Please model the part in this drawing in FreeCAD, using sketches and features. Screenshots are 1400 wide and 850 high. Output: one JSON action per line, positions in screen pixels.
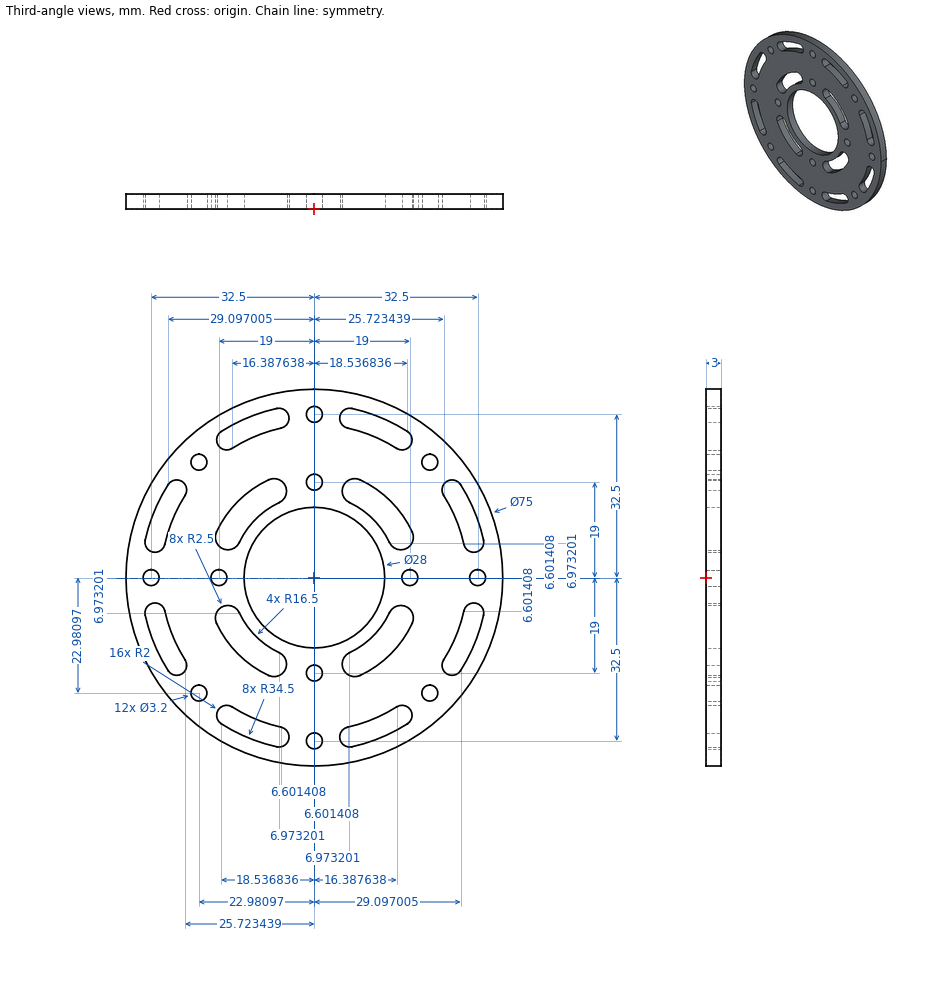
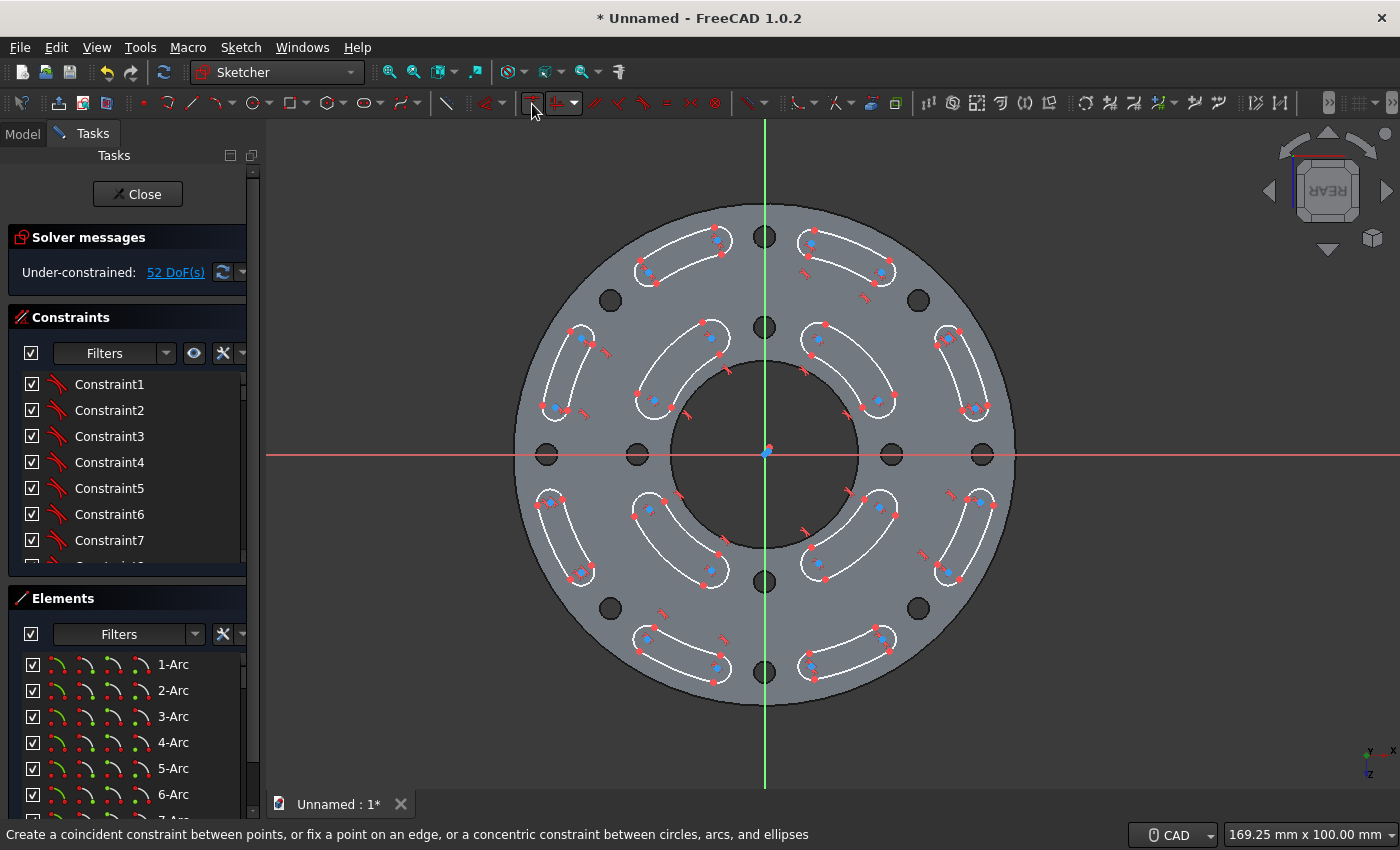
{"action": "left_click", "coordinate": [691, 235]}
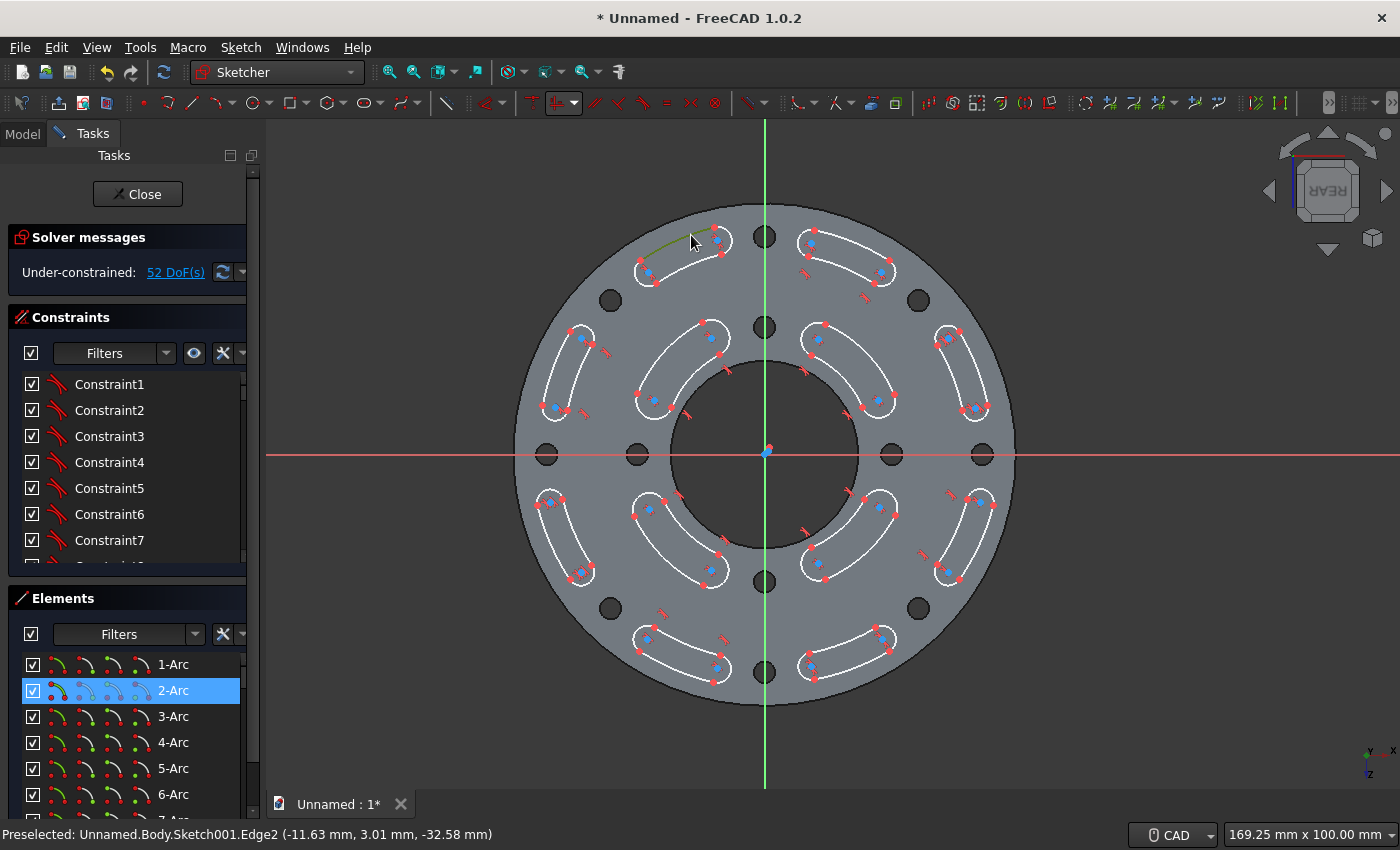
{"action": "left_click", "coordinate": [650, 542]}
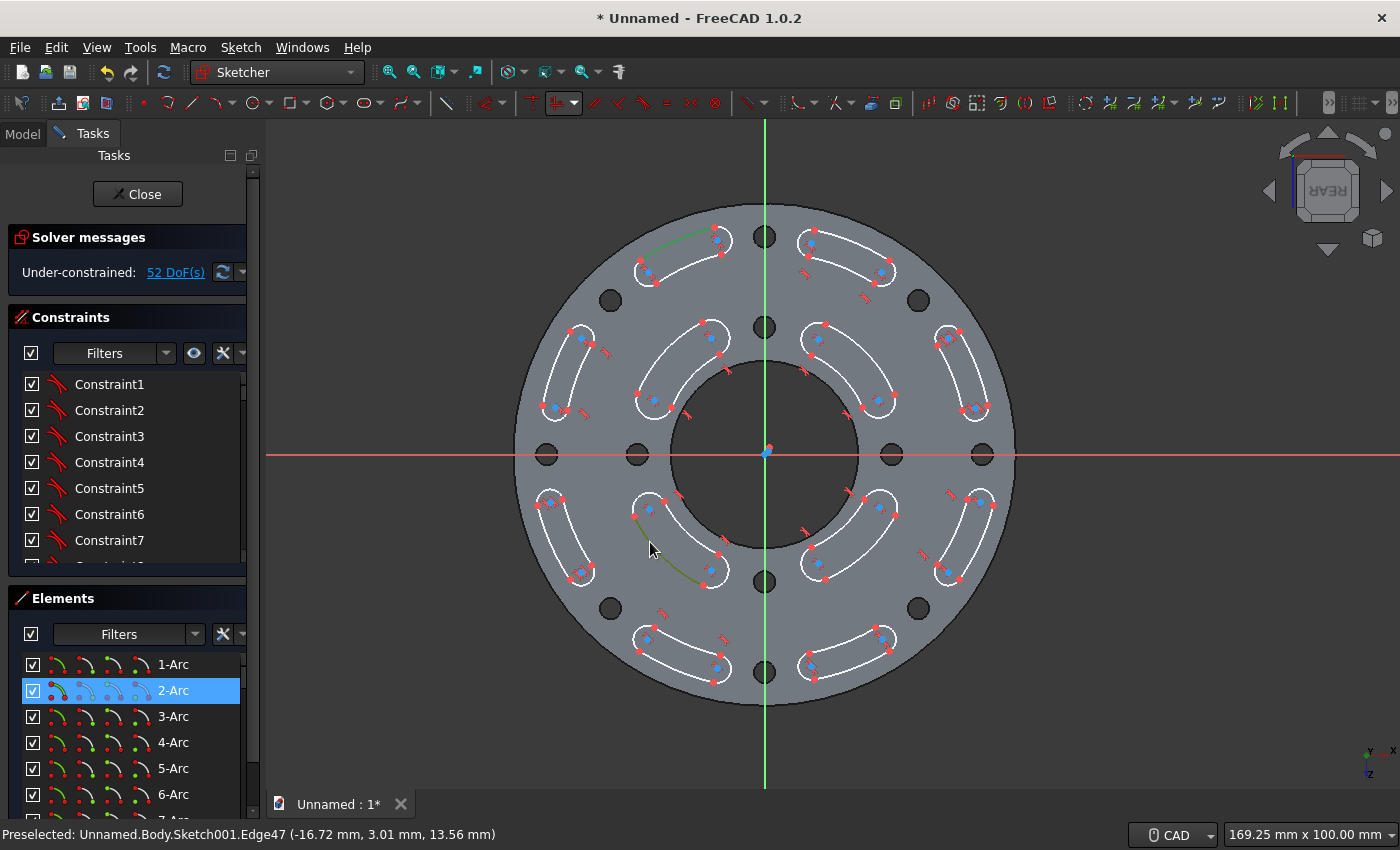
{"action": "left_click", "coordinate": [532, 104]}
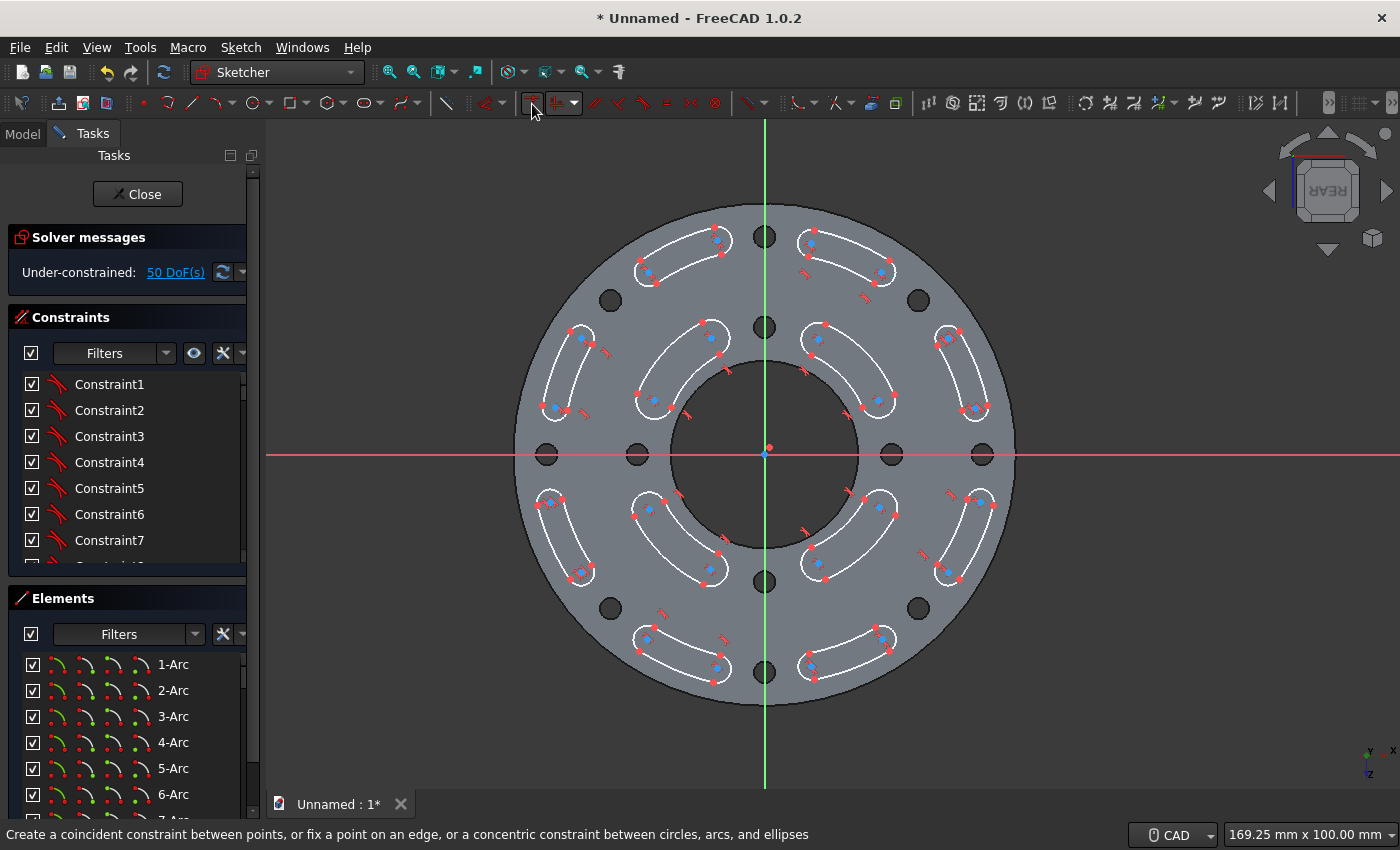
{"action": "scroll", "coordinate": [767, 451], "scroll_direction": "up", "scroll_amount": 6}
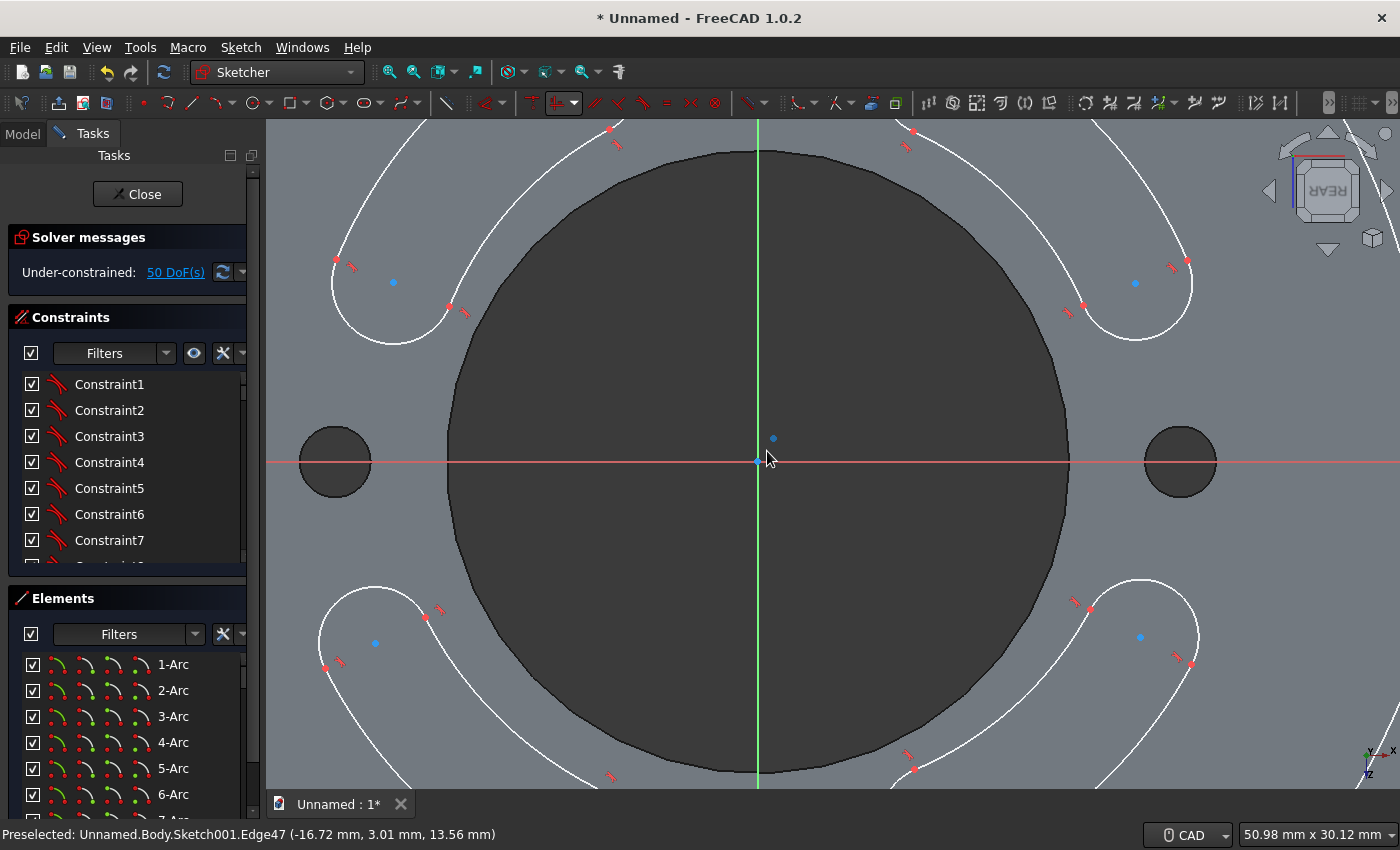
{"action": "left_click_drag", "start_coordinate": [748, 429], "coordinate": [784, 472]}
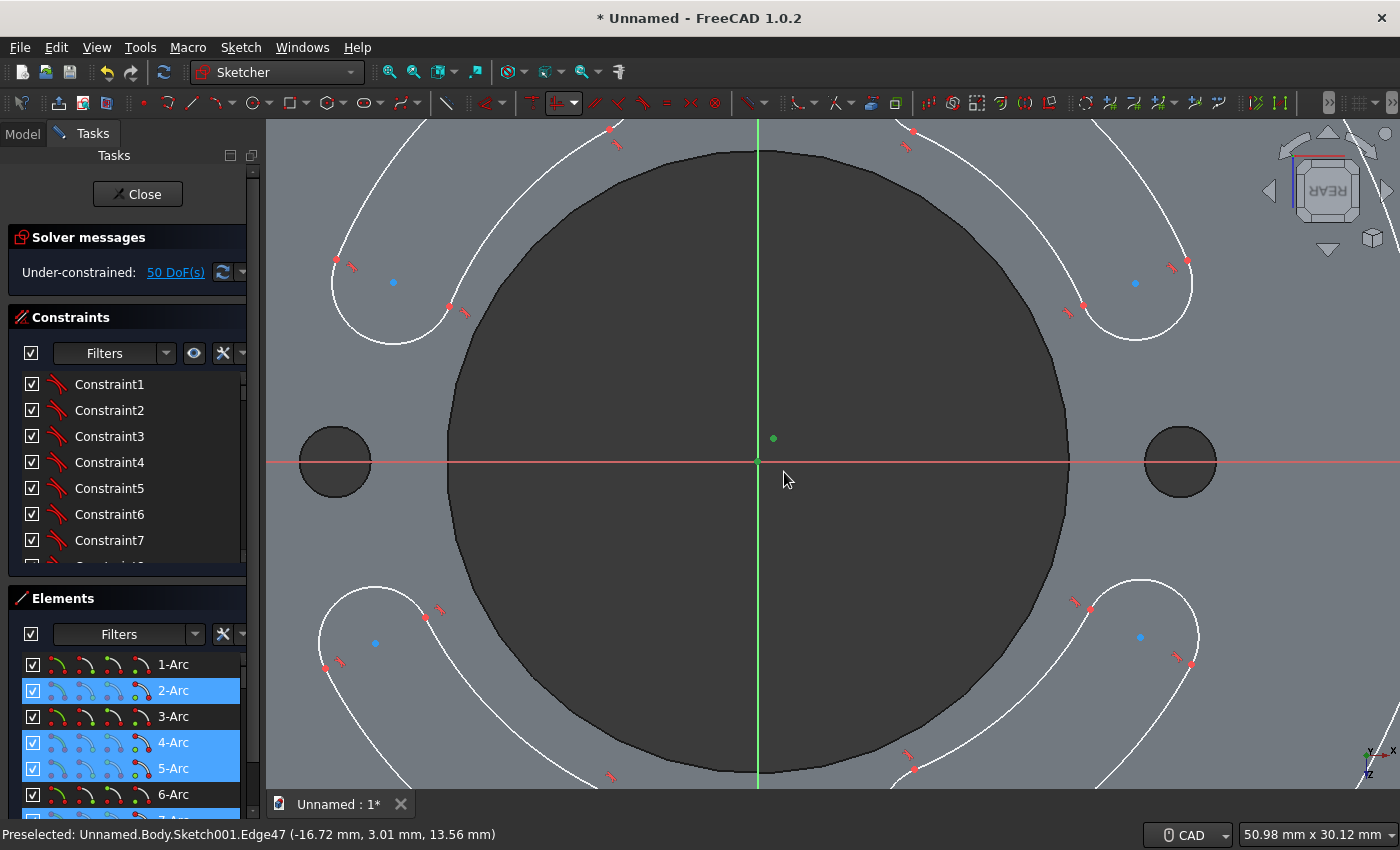
{"action": "left_click", "coordinate": [532, 104]}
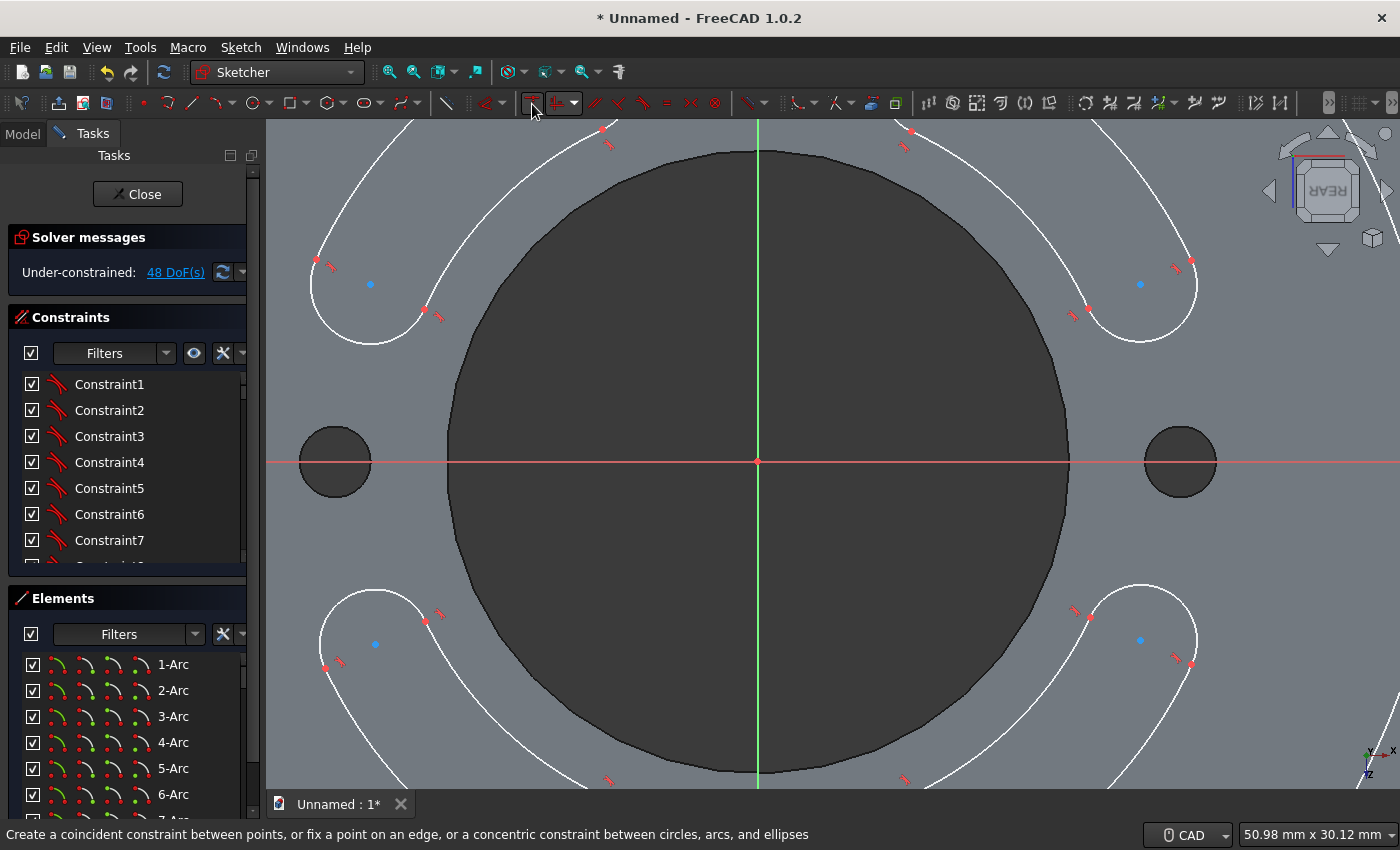
{"action": "scroll", "coordinate": [767, 451], "scroll_direction": "down", "scroll_amount": 6}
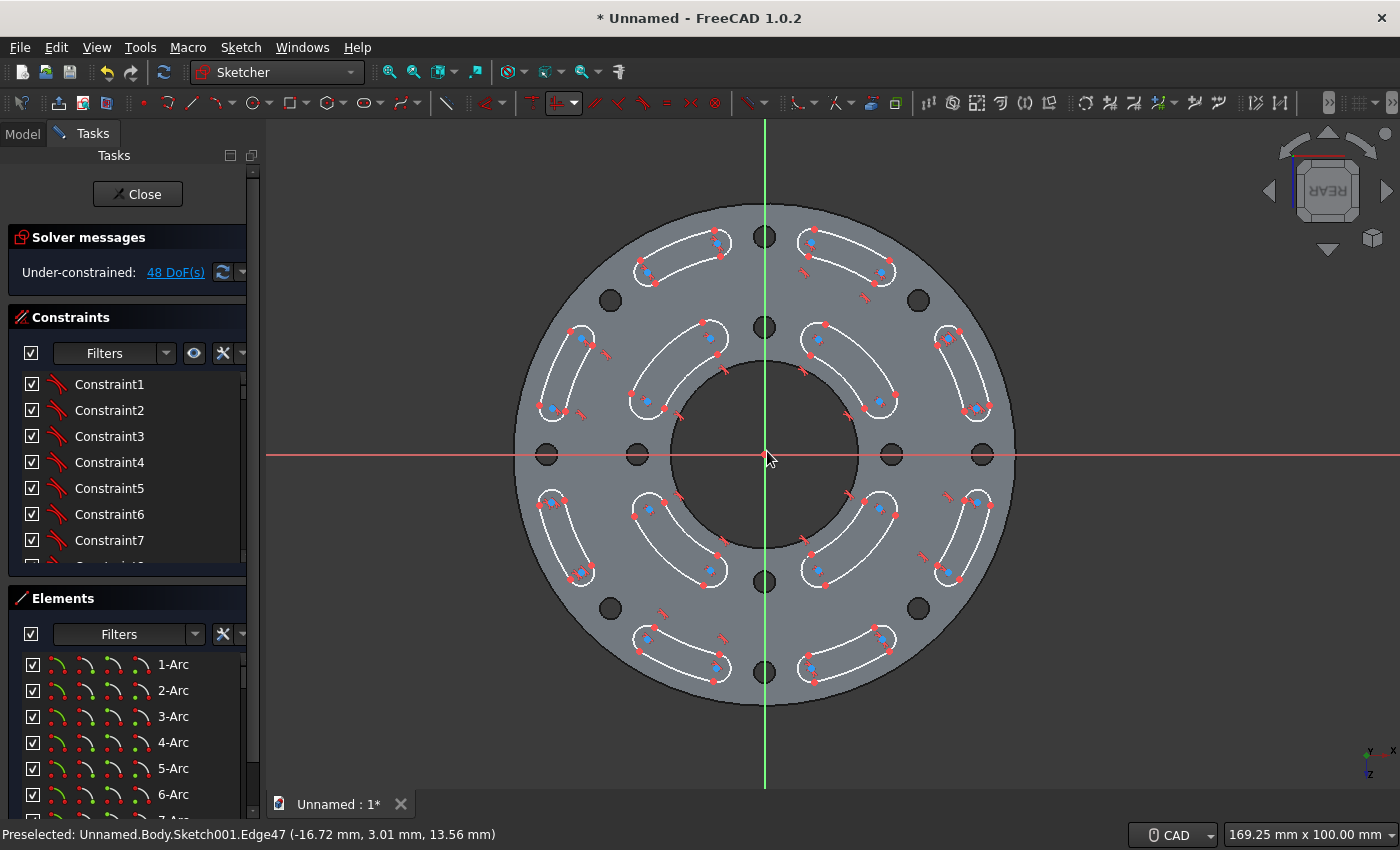
{"action": "left_click", "coordinate": [700, 262]}